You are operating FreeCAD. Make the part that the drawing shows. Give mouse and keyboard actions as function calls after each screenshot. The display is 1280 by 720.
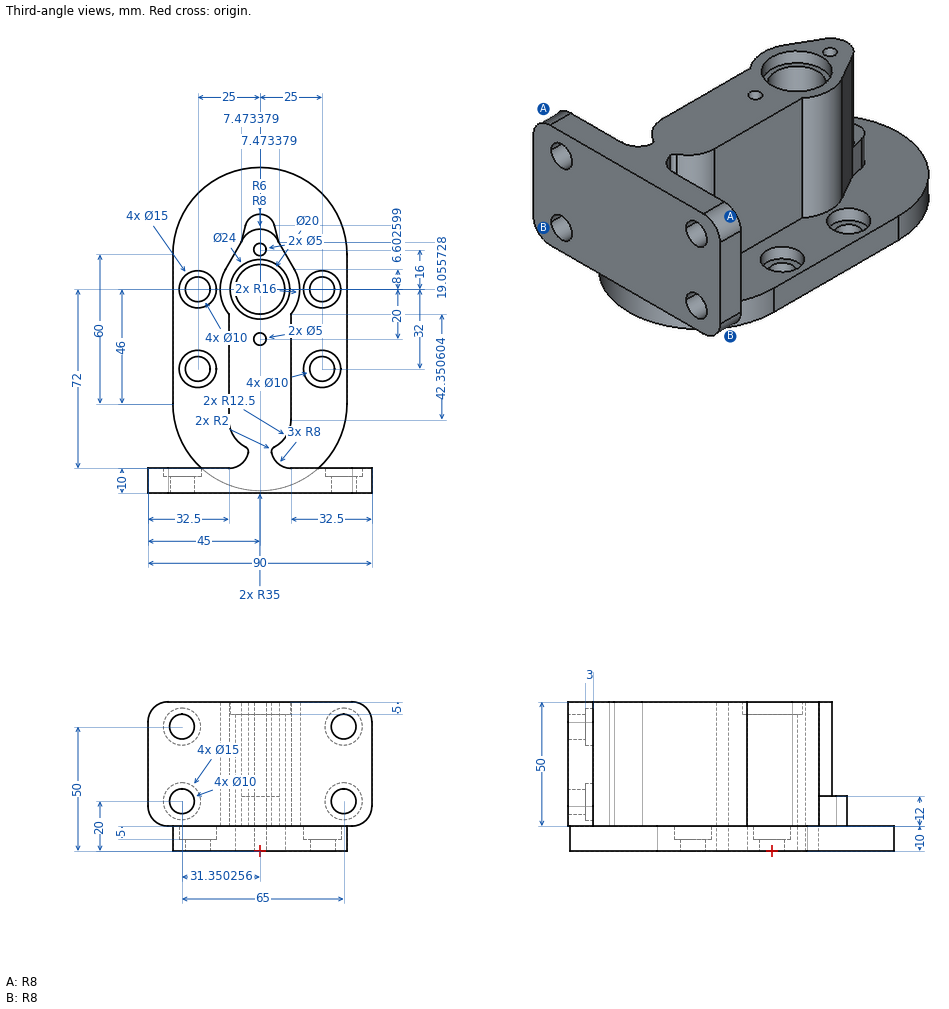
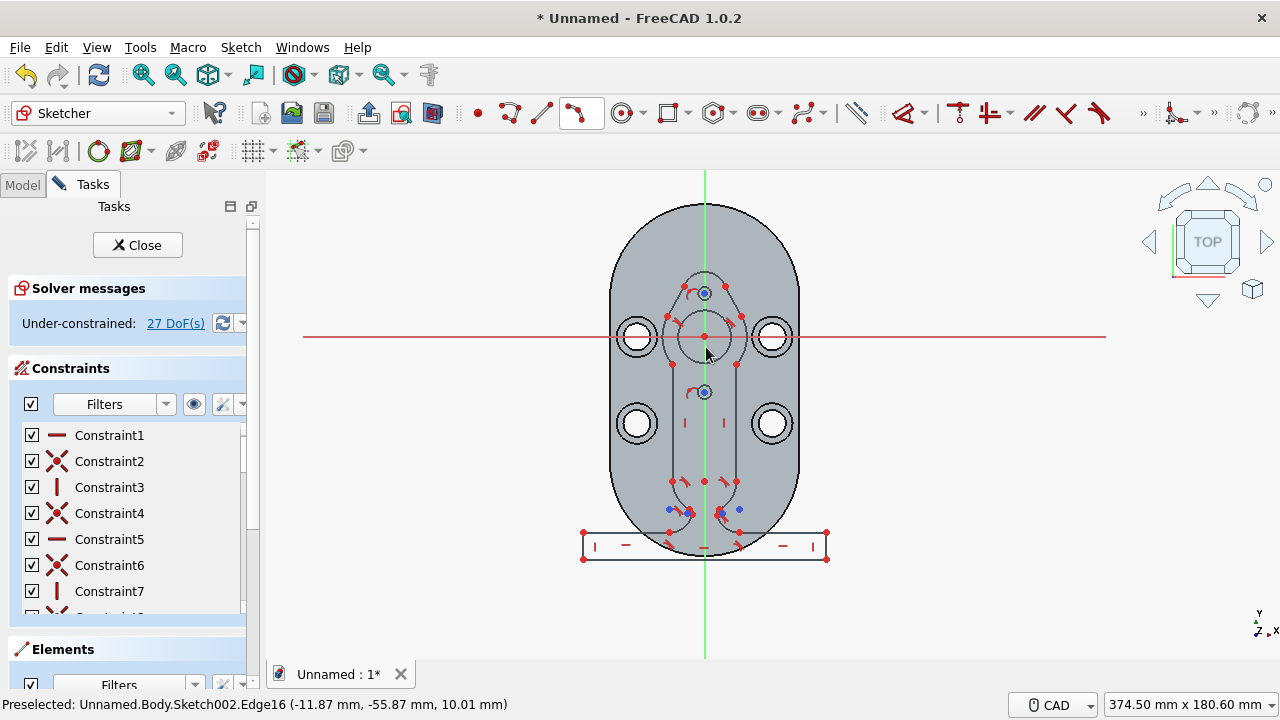
scroll(721, 524, up, 3)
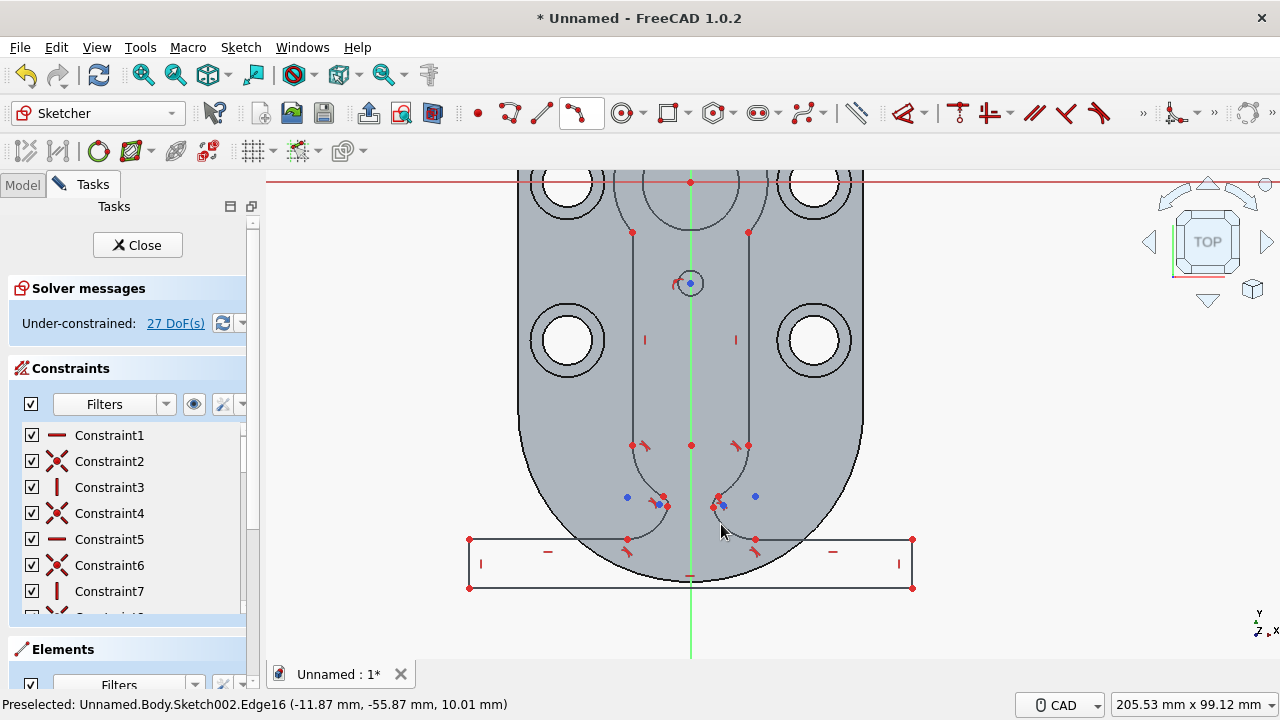
click(721, 523)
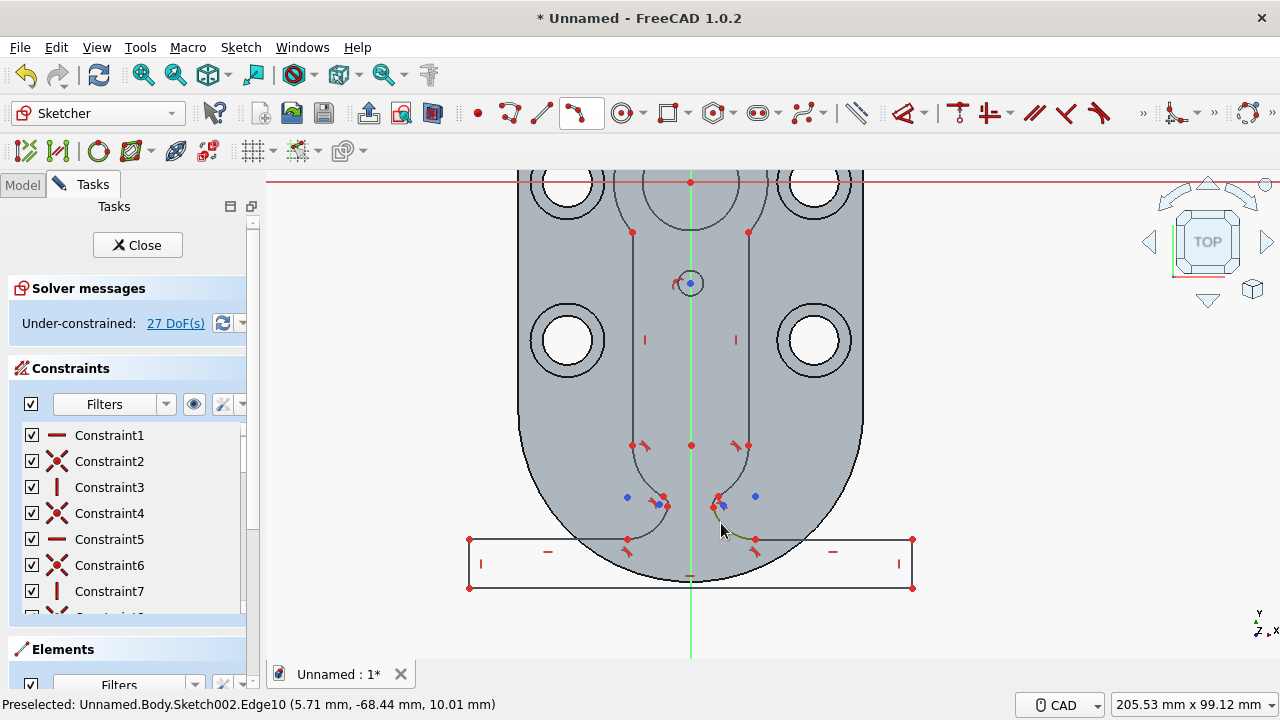
scroll(721, 523, down, 3)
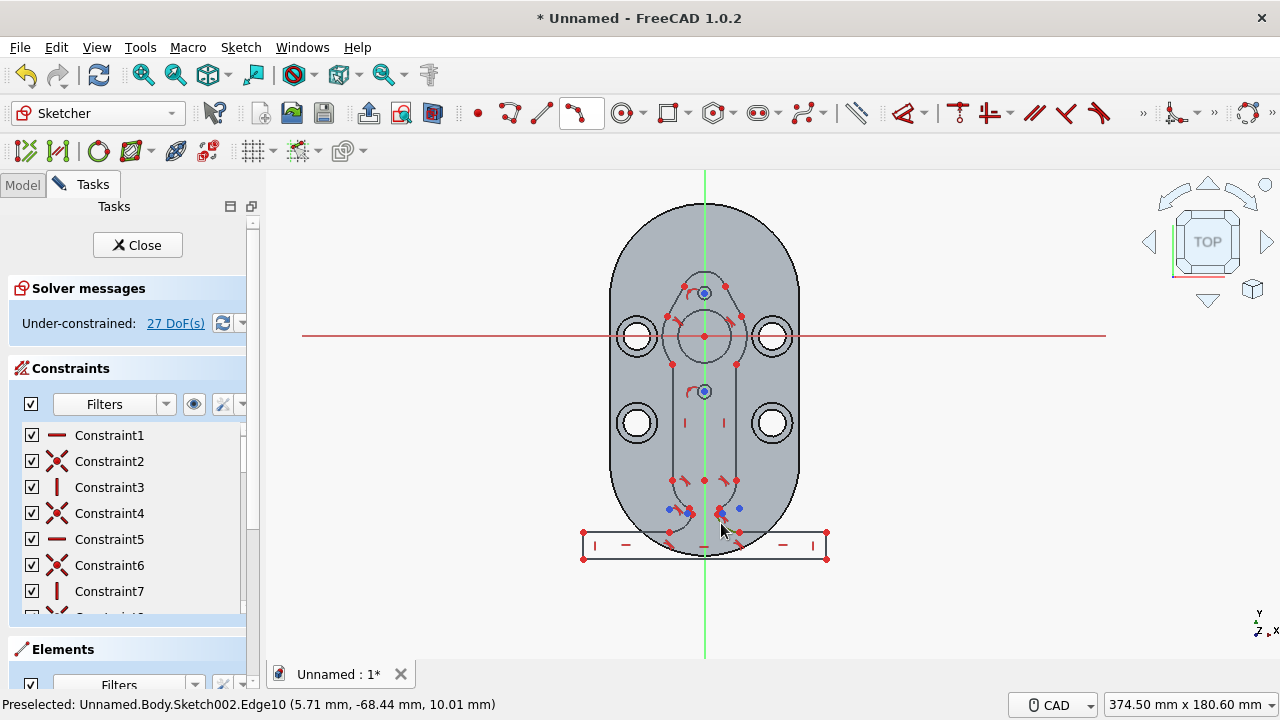
scroll(715, 274, up, 2)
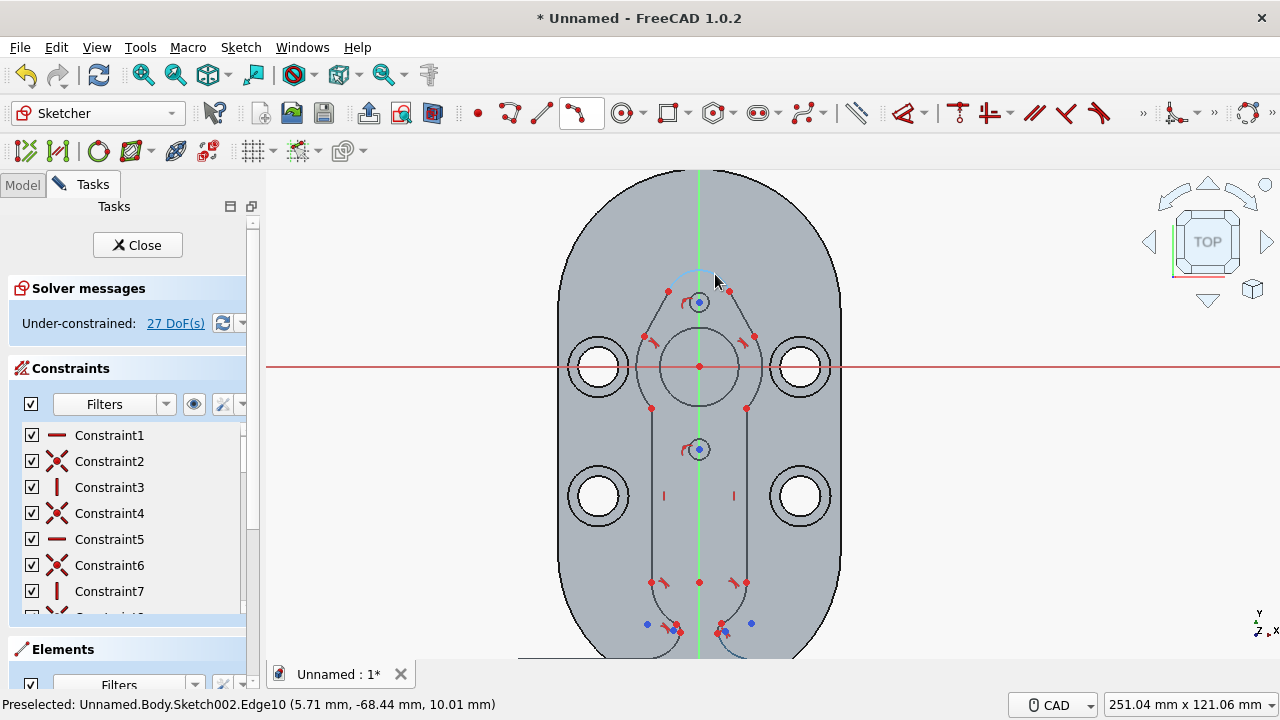
click(715, 274)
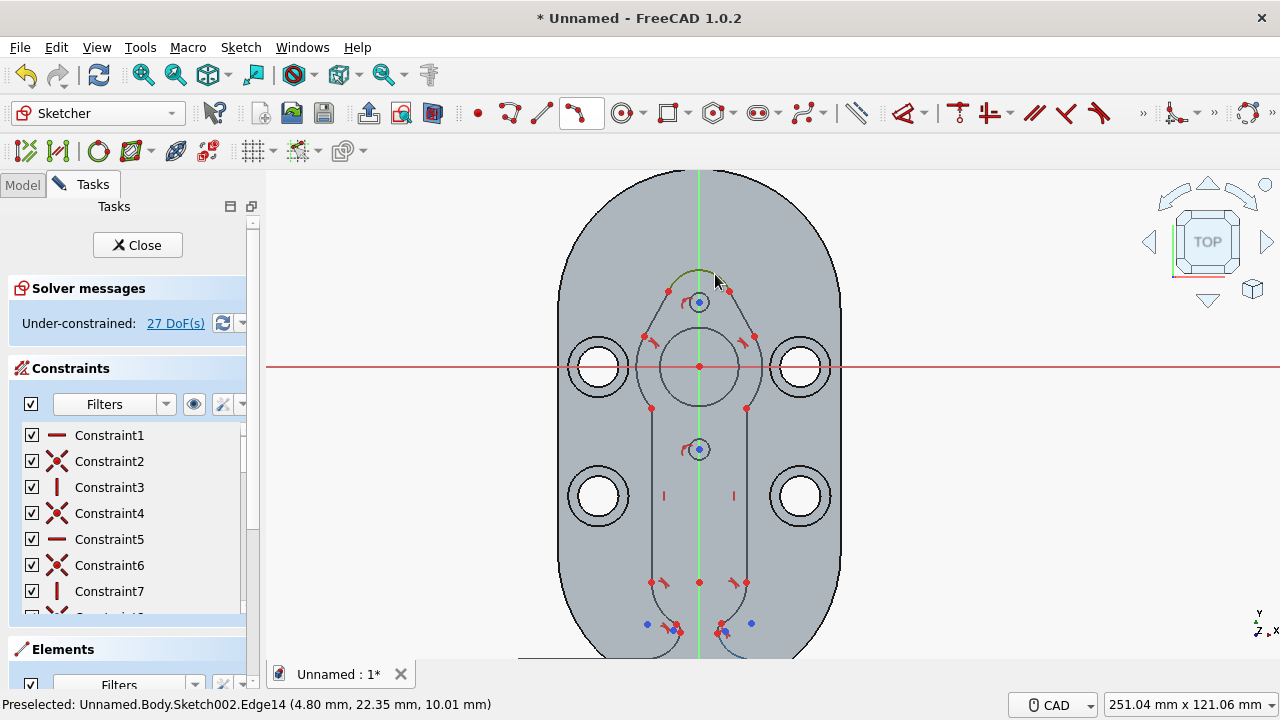
scroll(715, 274, down, 2)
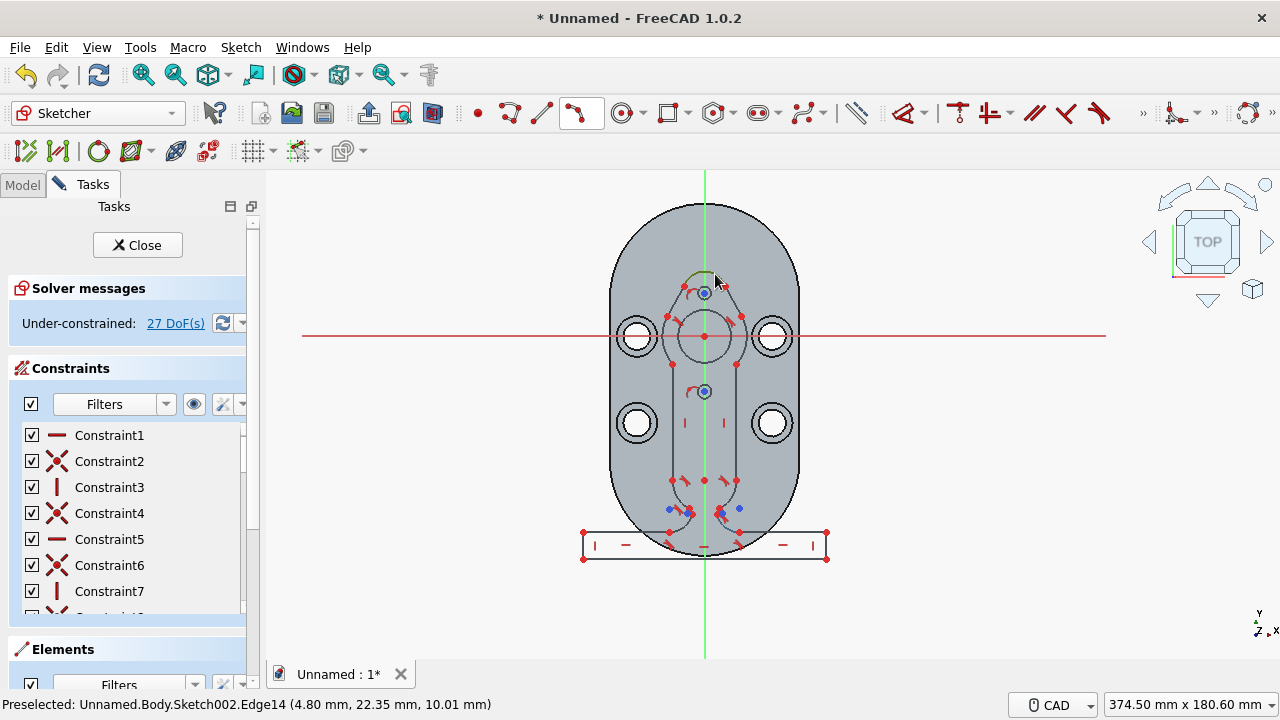
scroll(679, 530, up, 3)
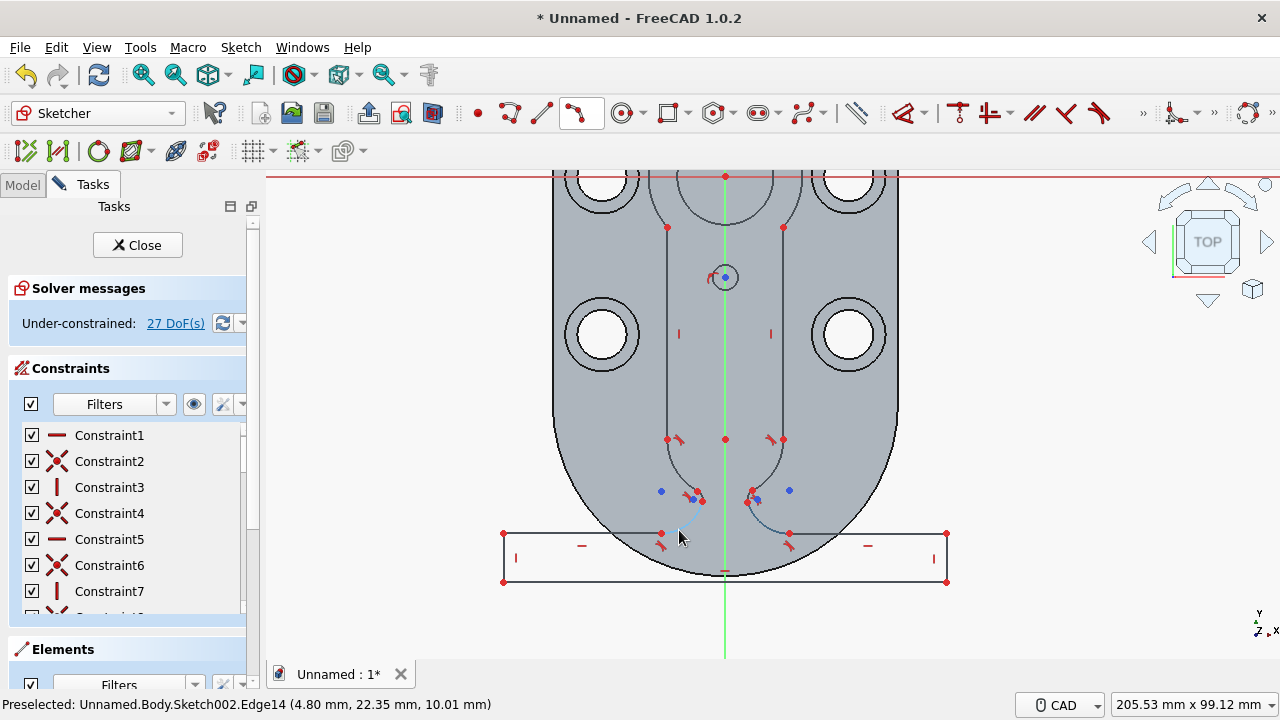
click(678, 530)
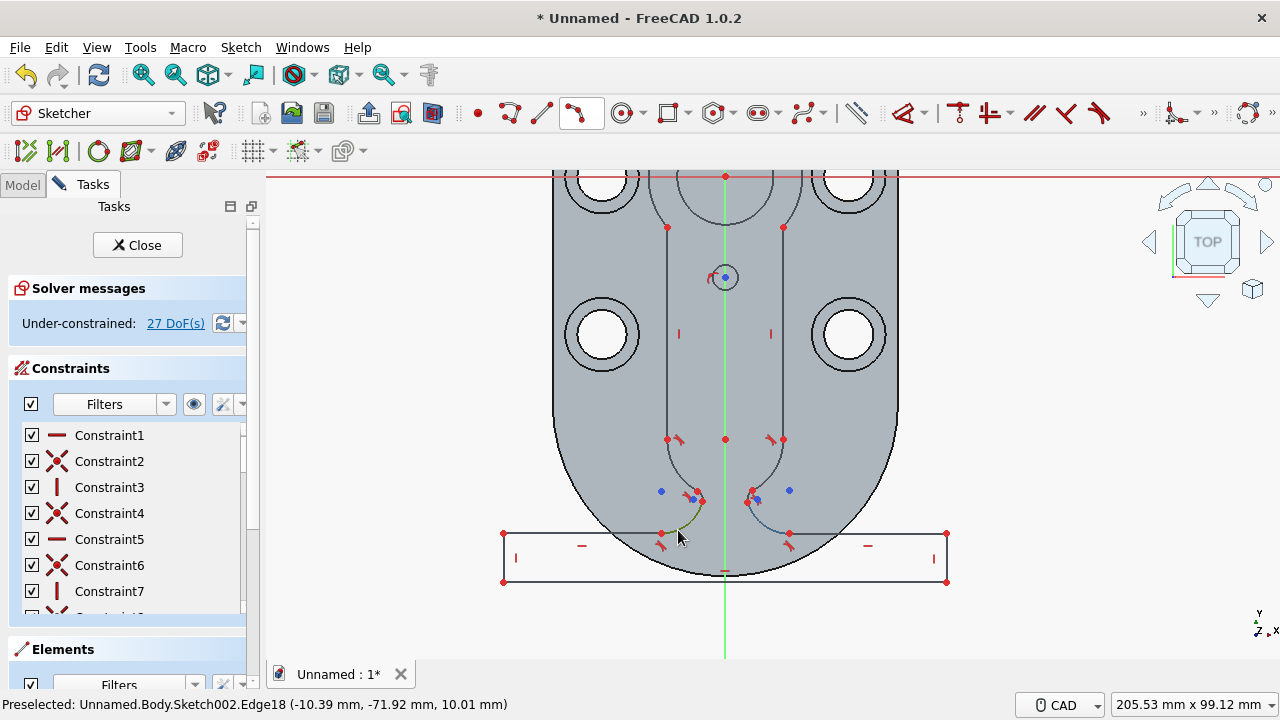
key(e)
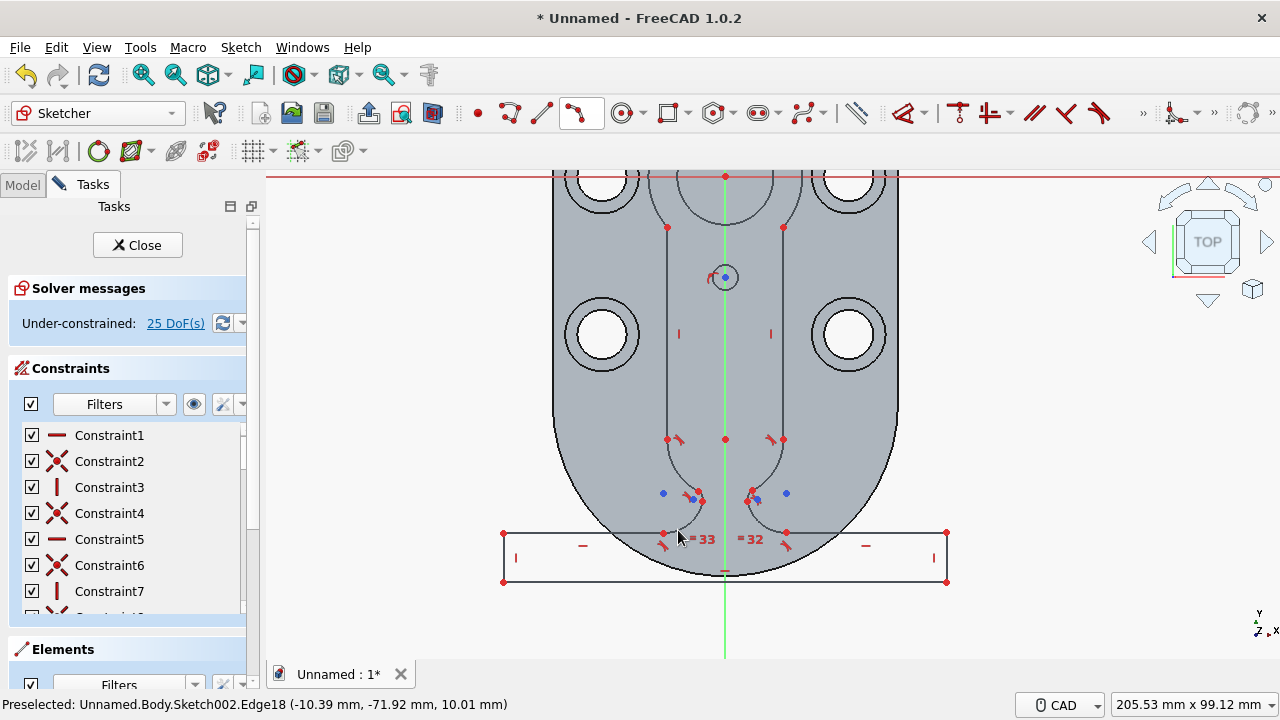
click(798, 203)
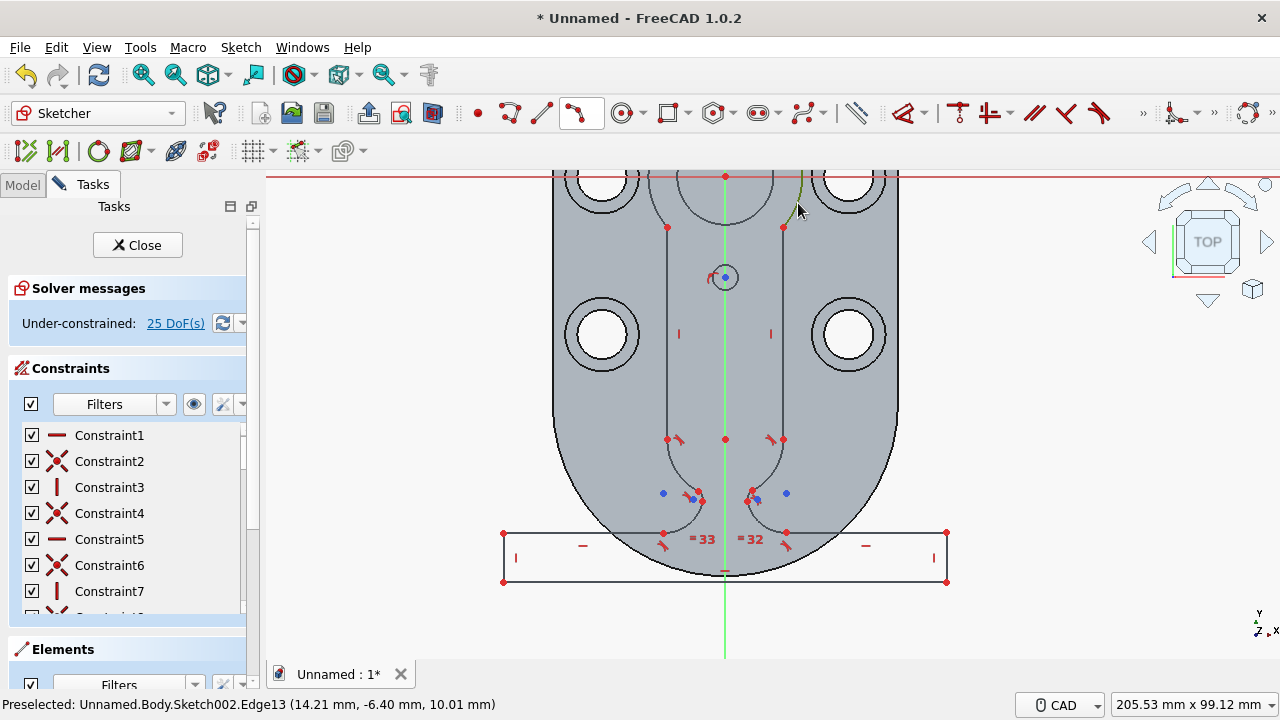
click(653, 203)